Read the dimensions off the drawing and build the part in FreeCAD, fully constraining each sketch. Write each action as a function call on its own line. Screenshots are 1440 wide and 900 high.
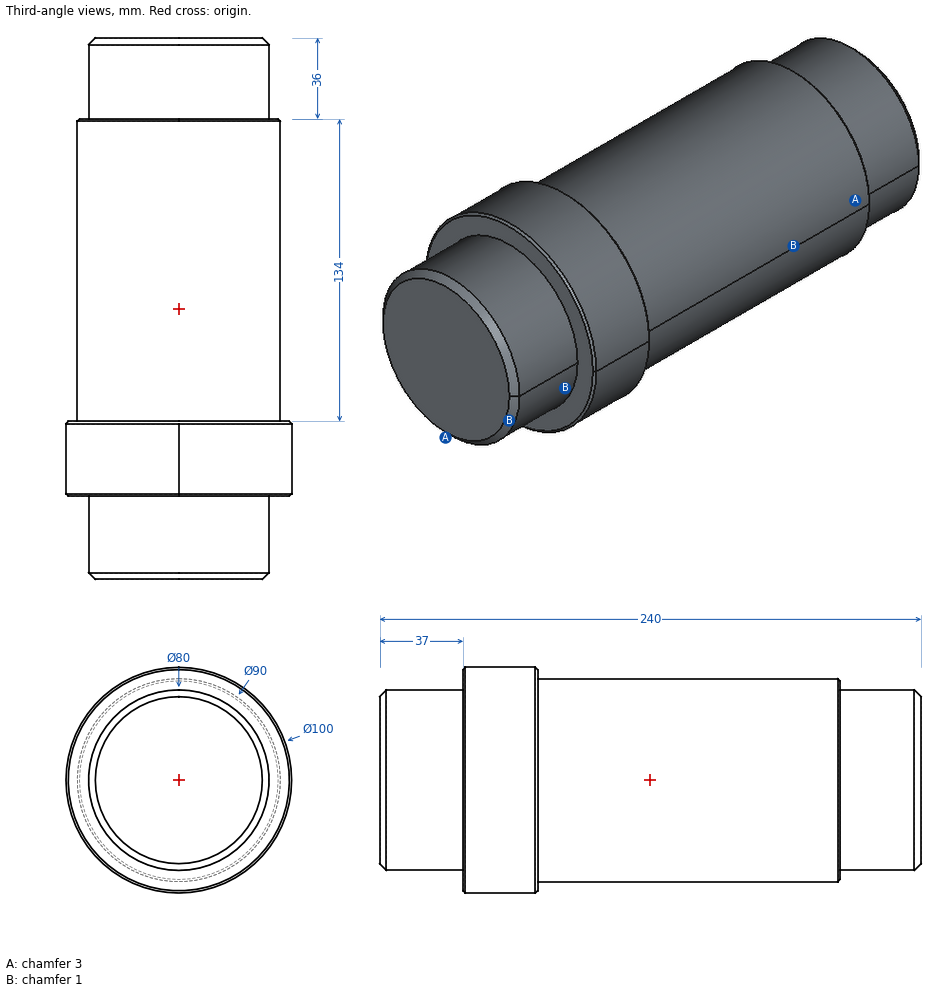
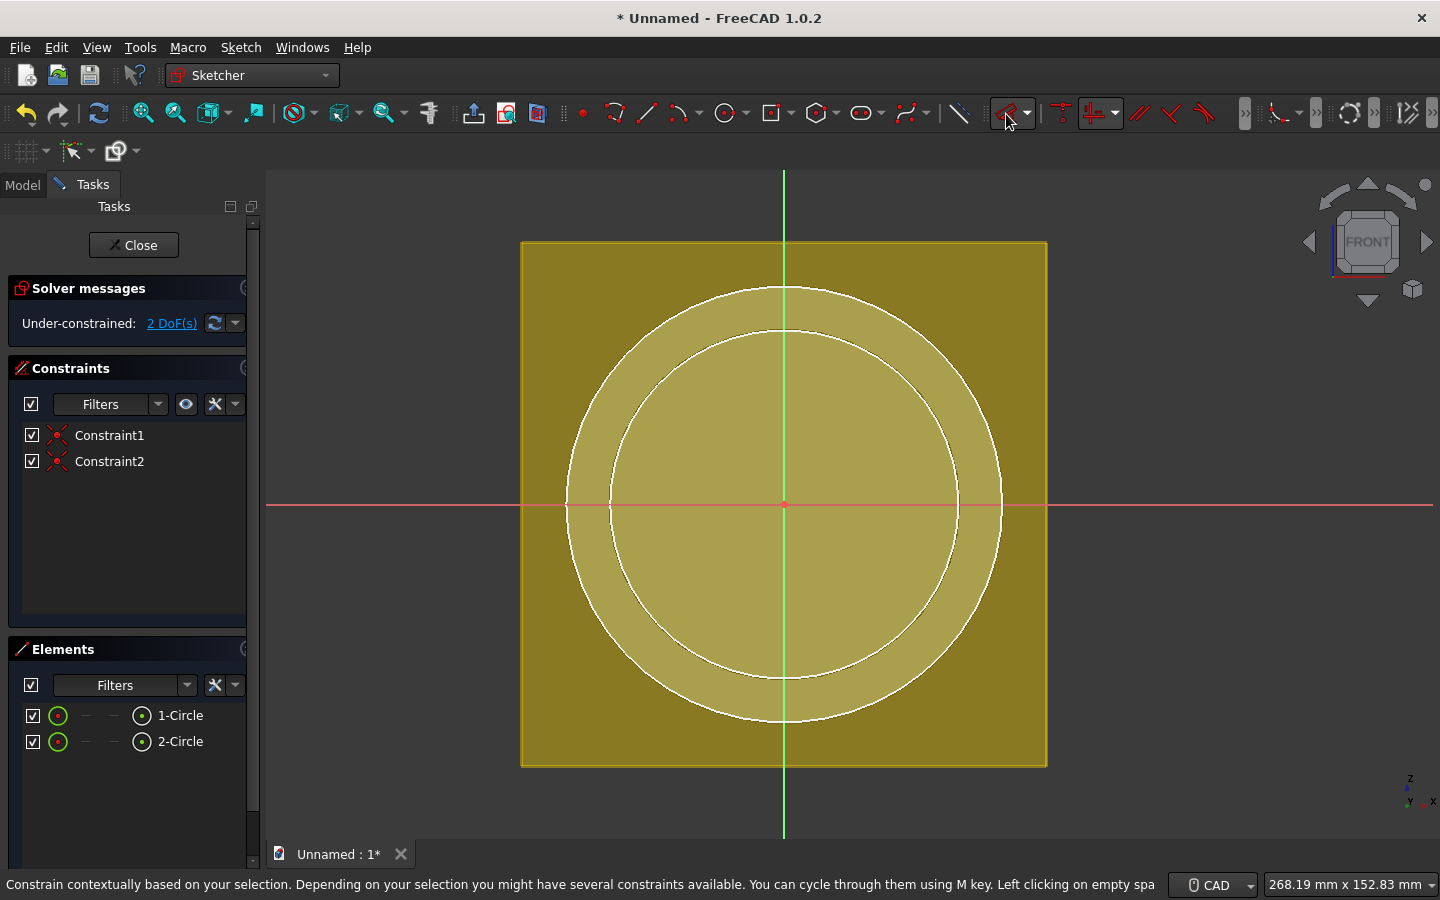
click(938, 350)
click(961, 327)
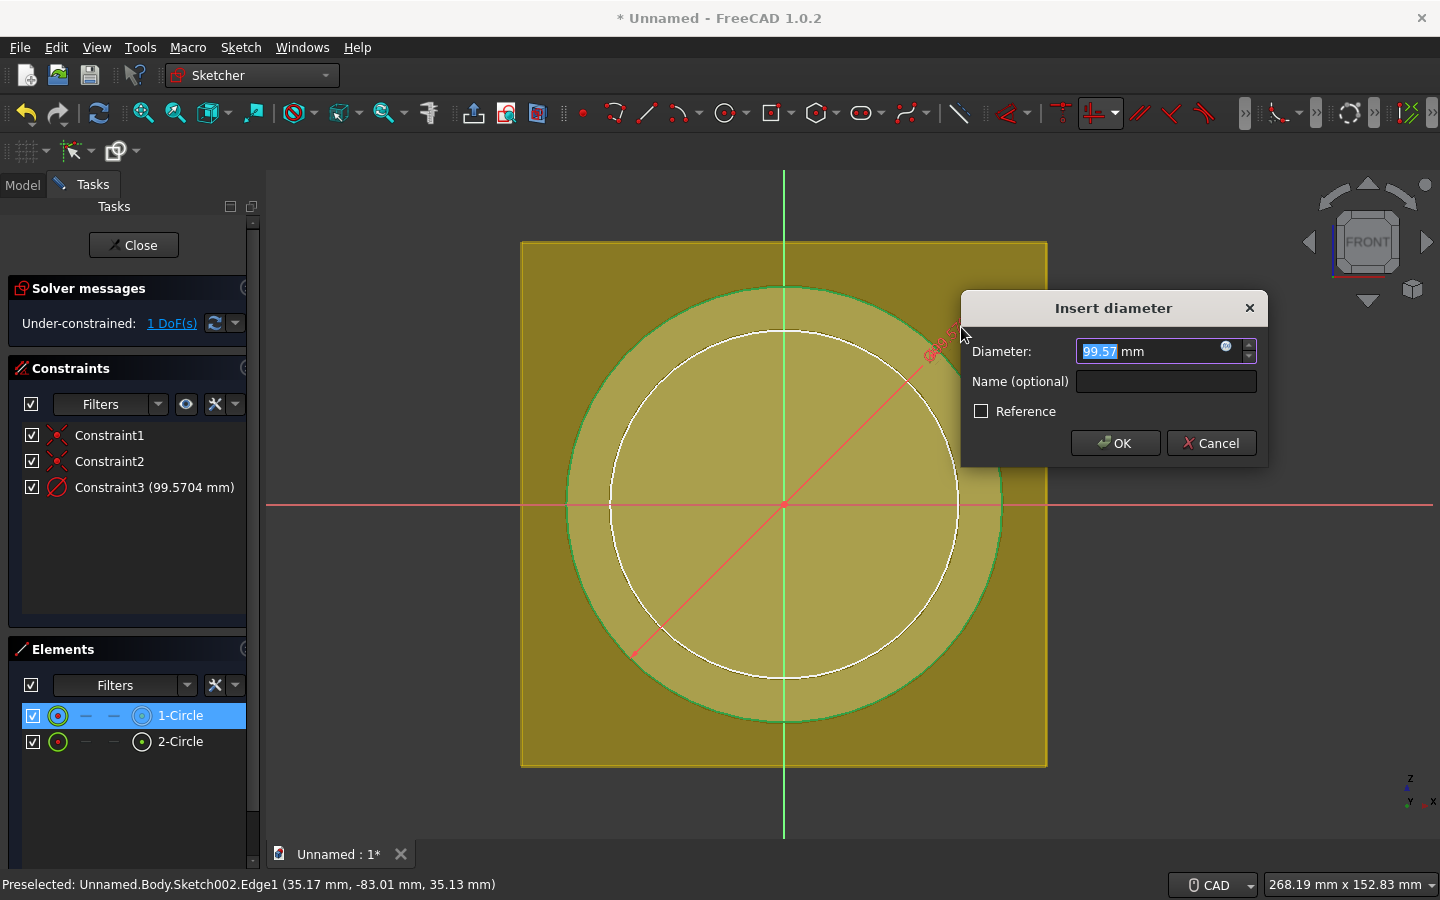
text(100)
key(Return)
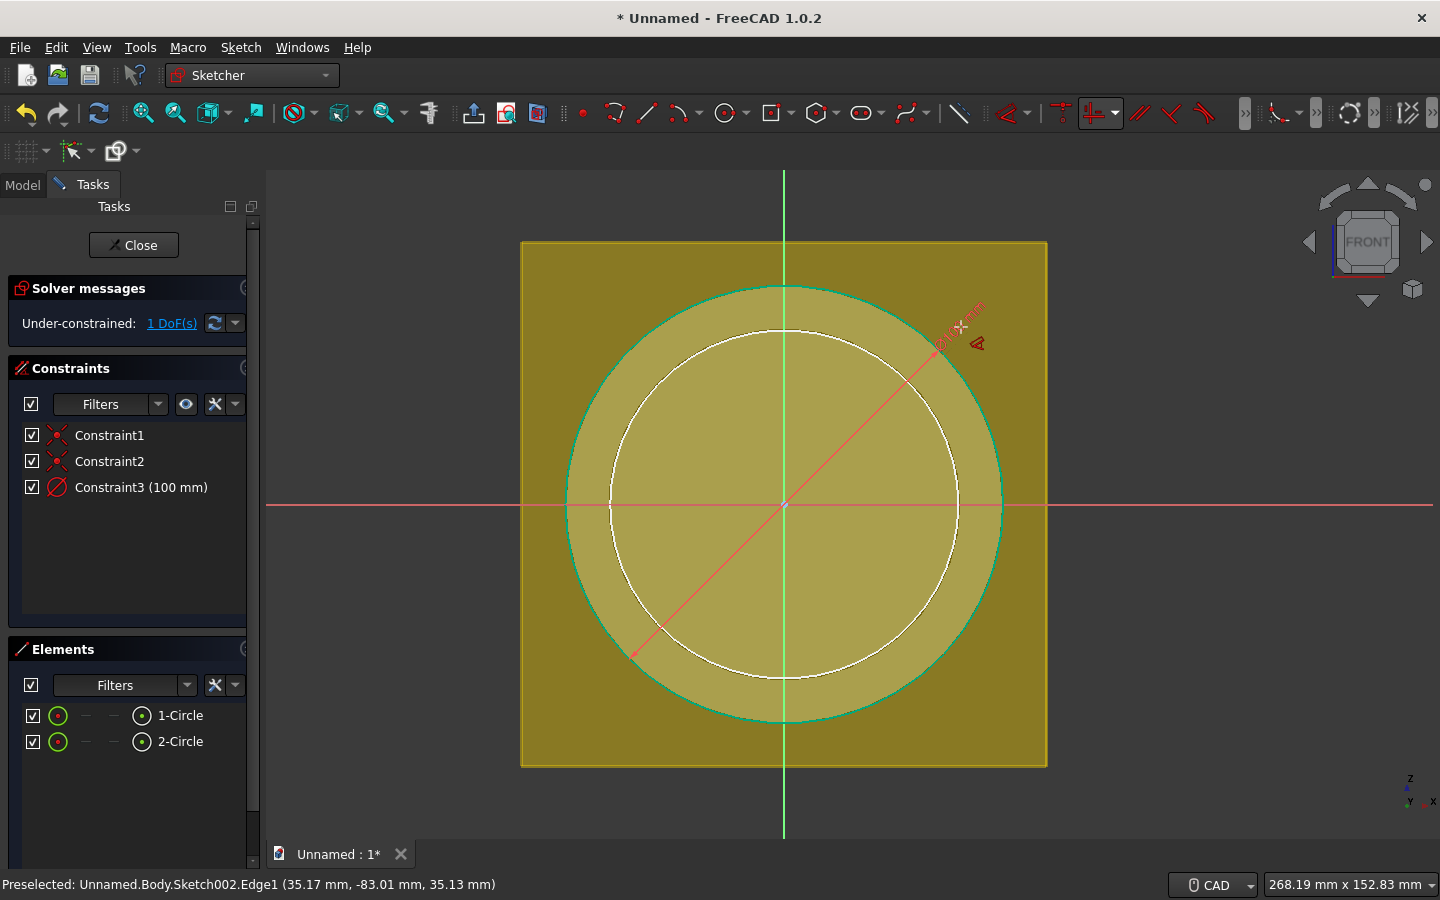
click(907, 381)
click(1028, 432)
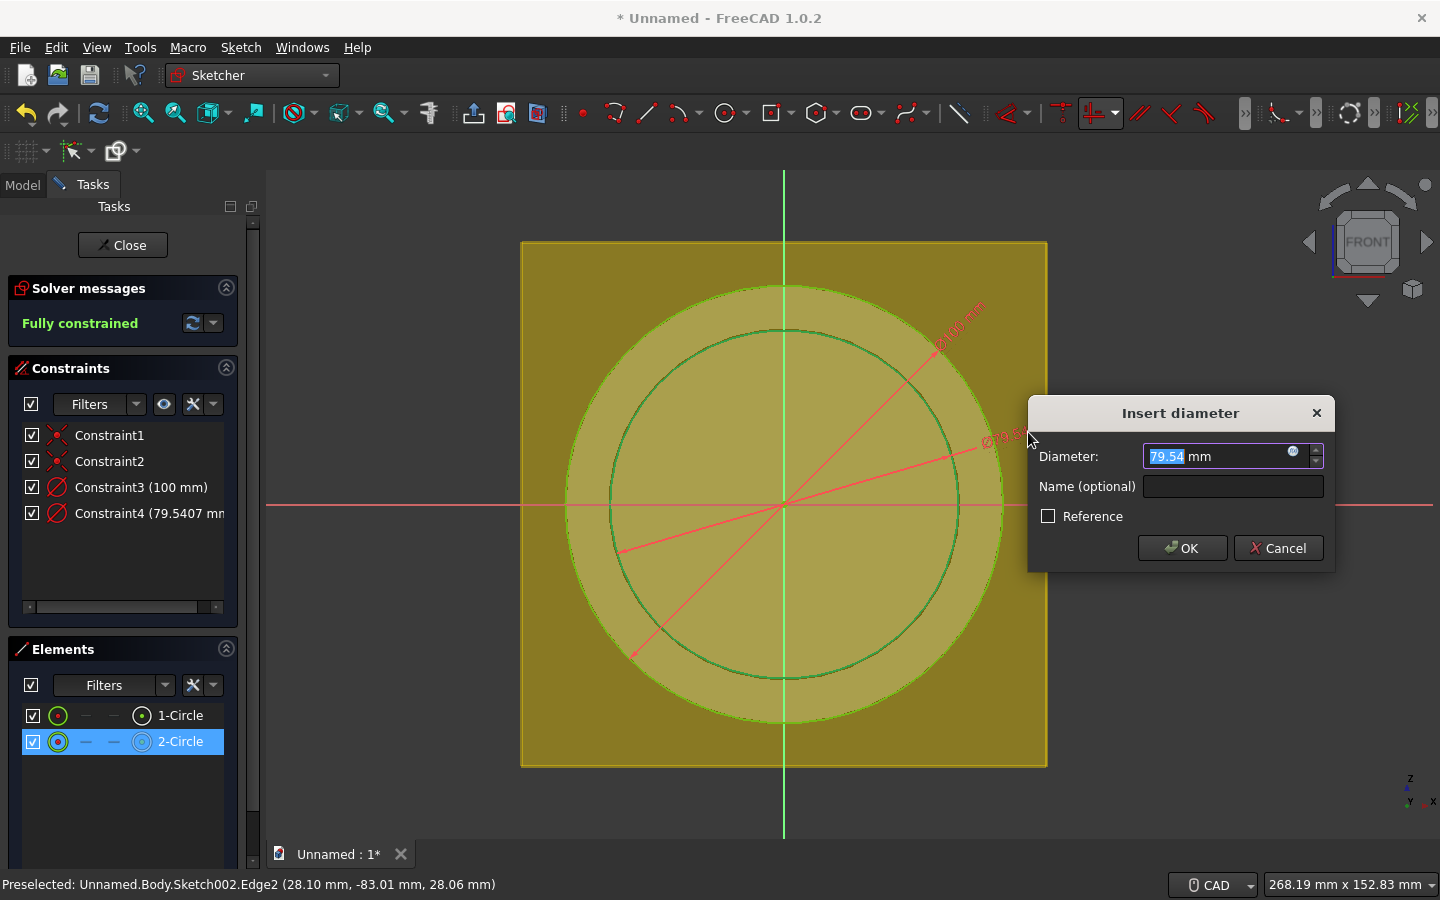
text(80)
key(Return)
key(Escape)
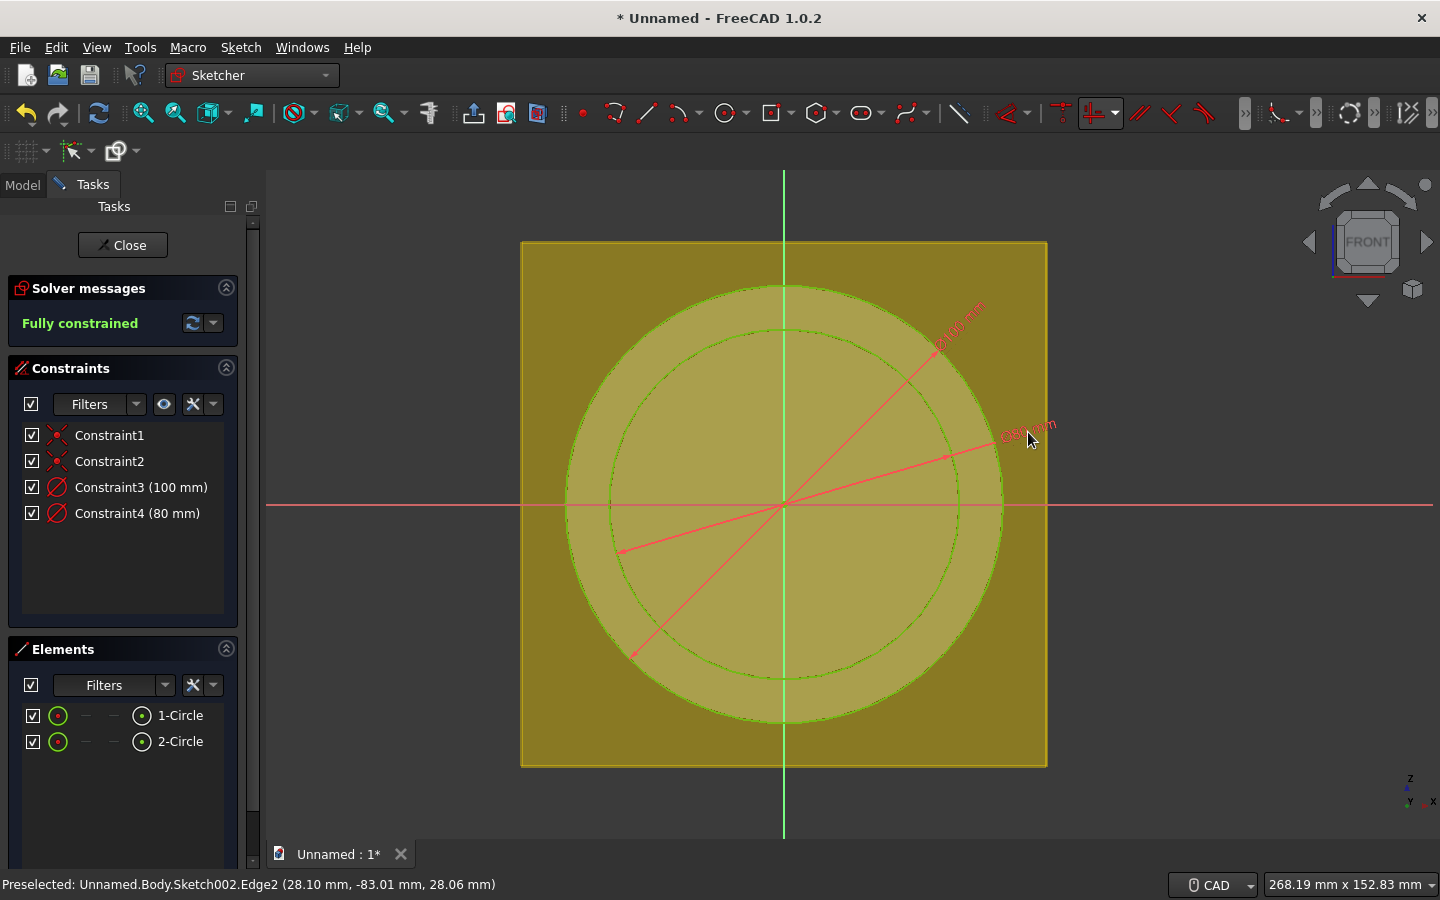
click(123, 245)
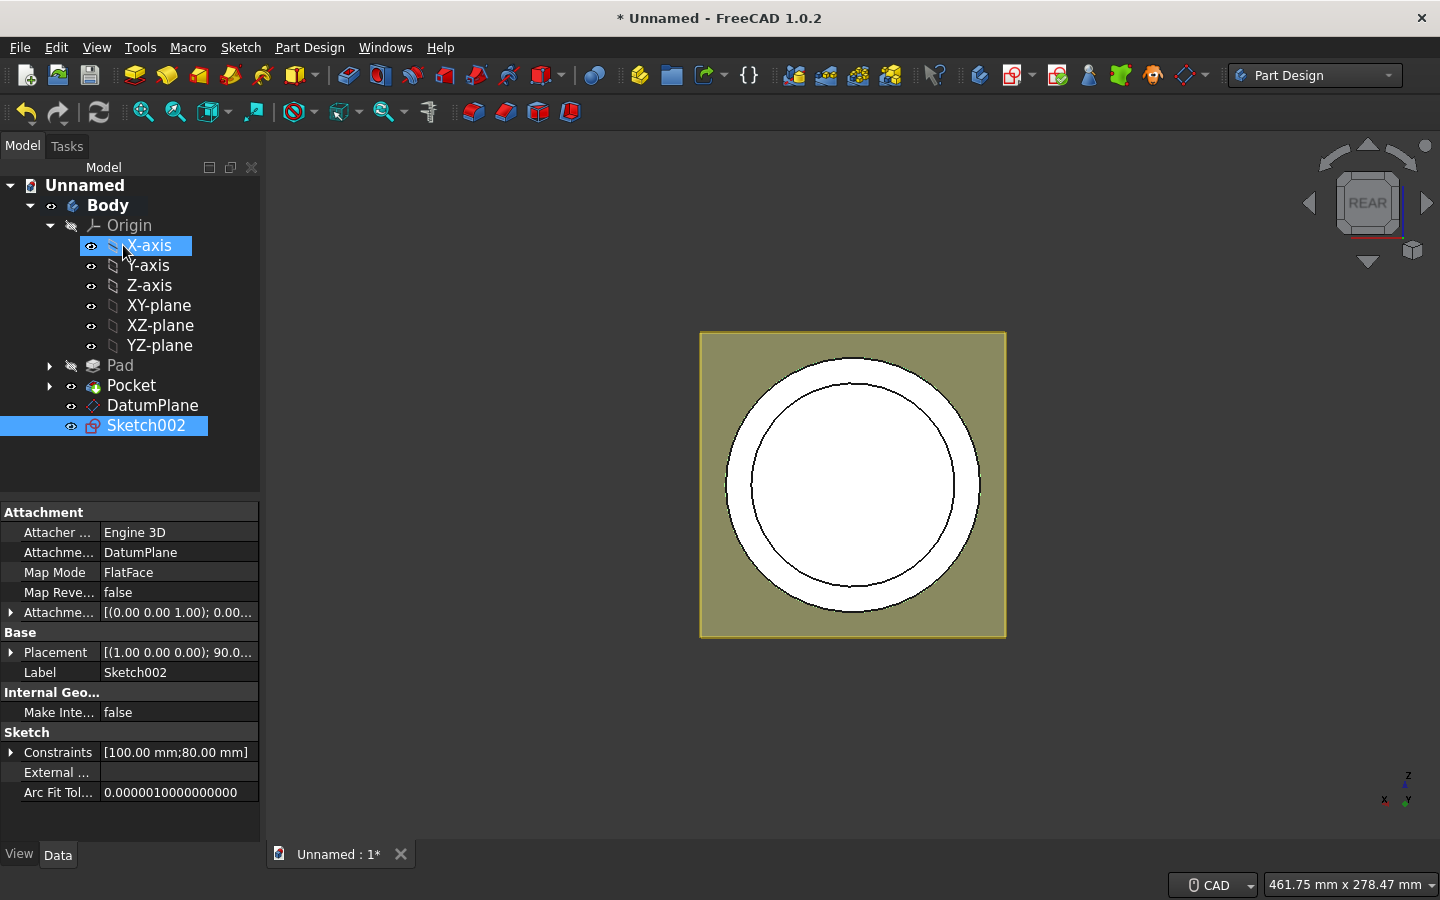
click(350, 76)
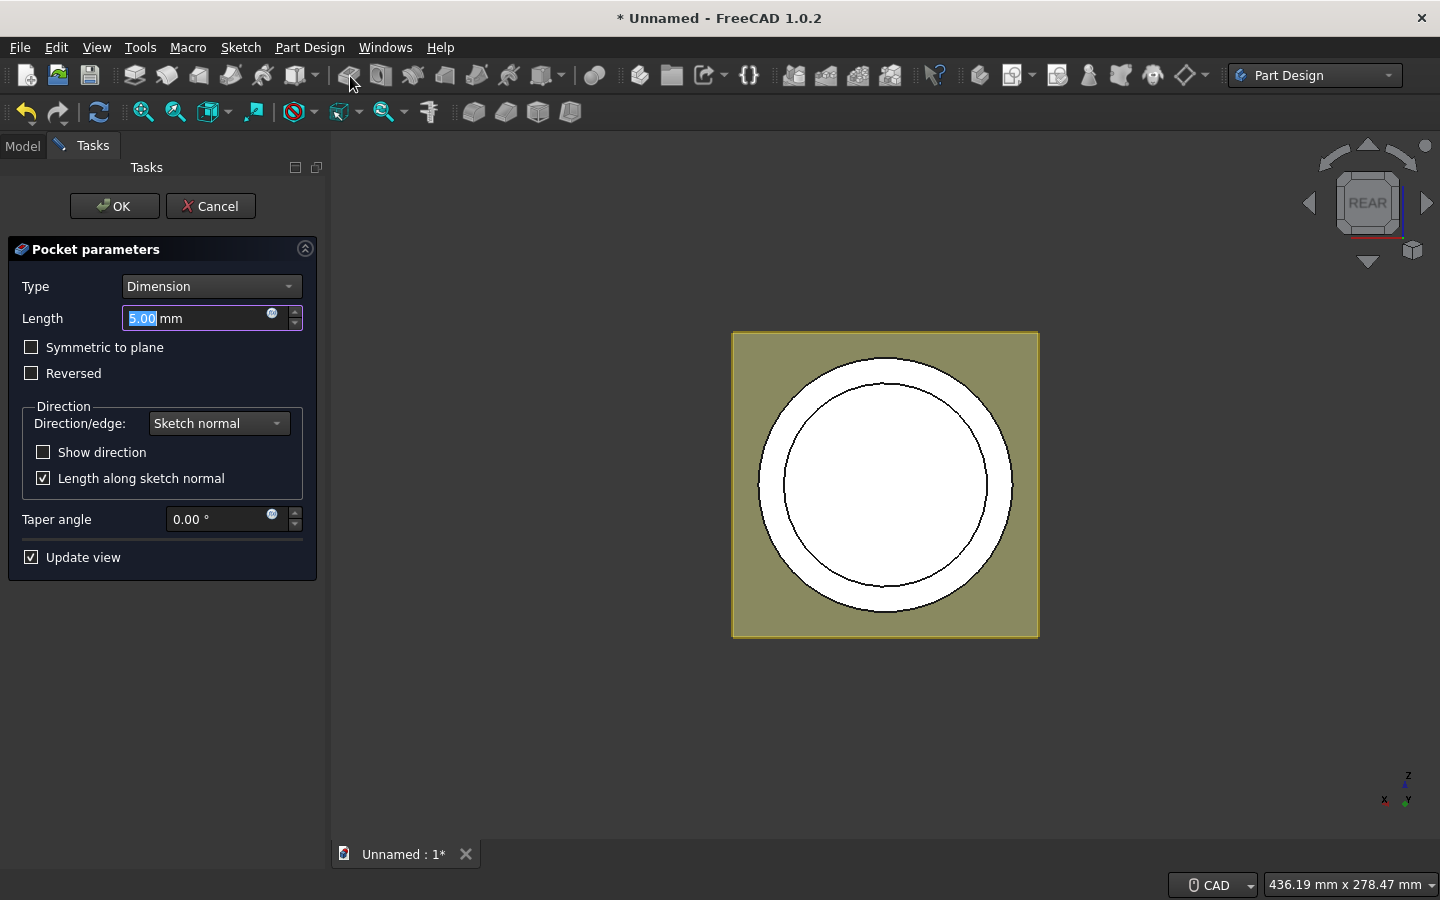
text(37)
key(Tab)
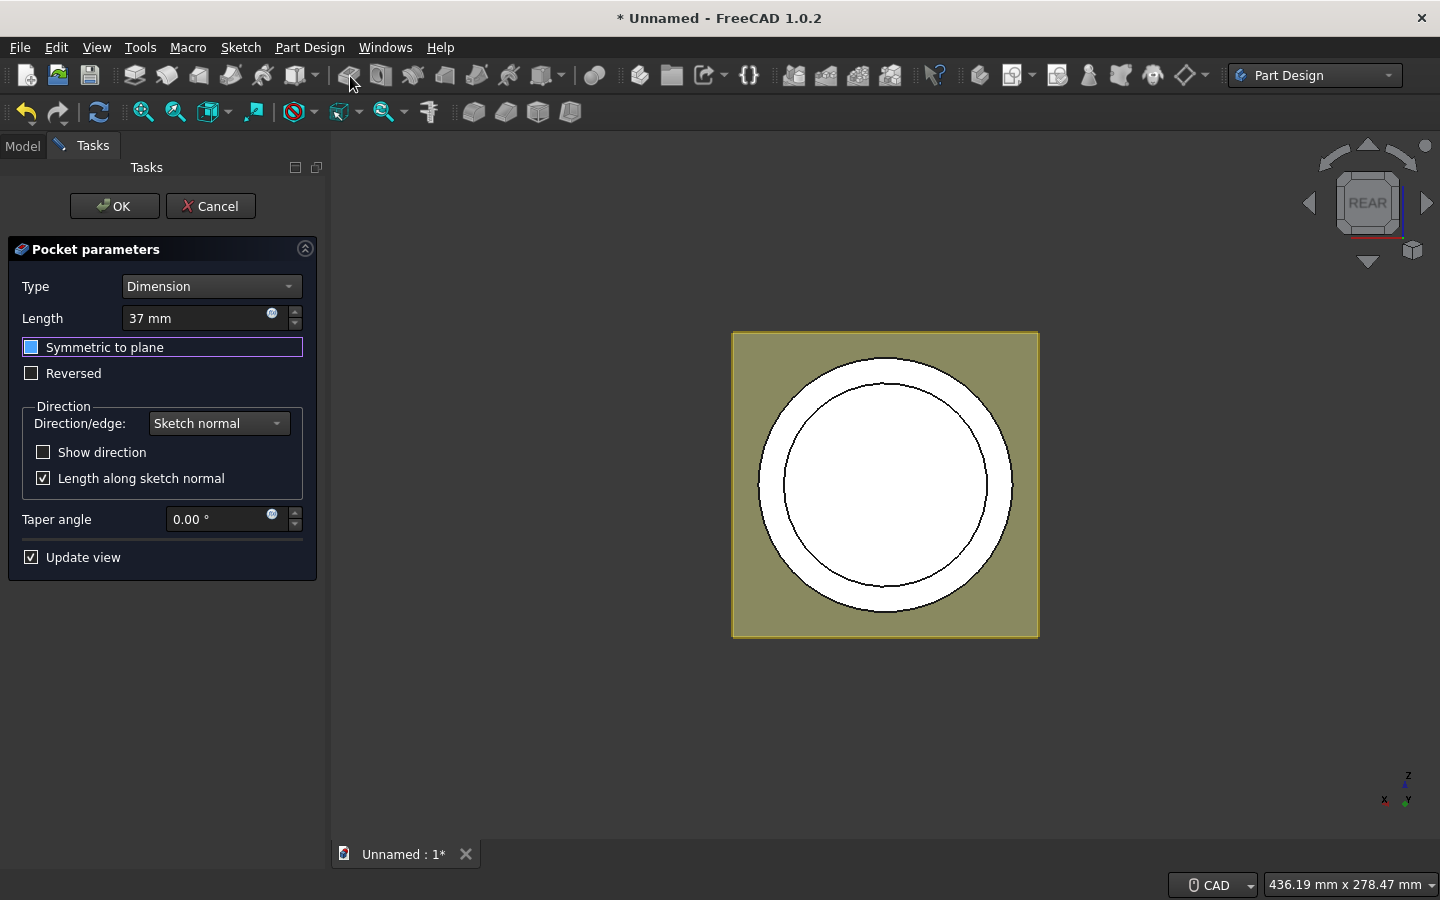
click(30, 373)